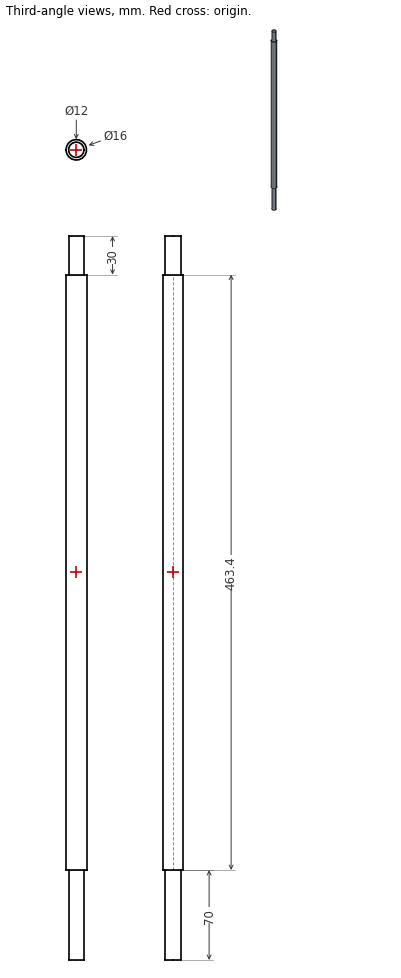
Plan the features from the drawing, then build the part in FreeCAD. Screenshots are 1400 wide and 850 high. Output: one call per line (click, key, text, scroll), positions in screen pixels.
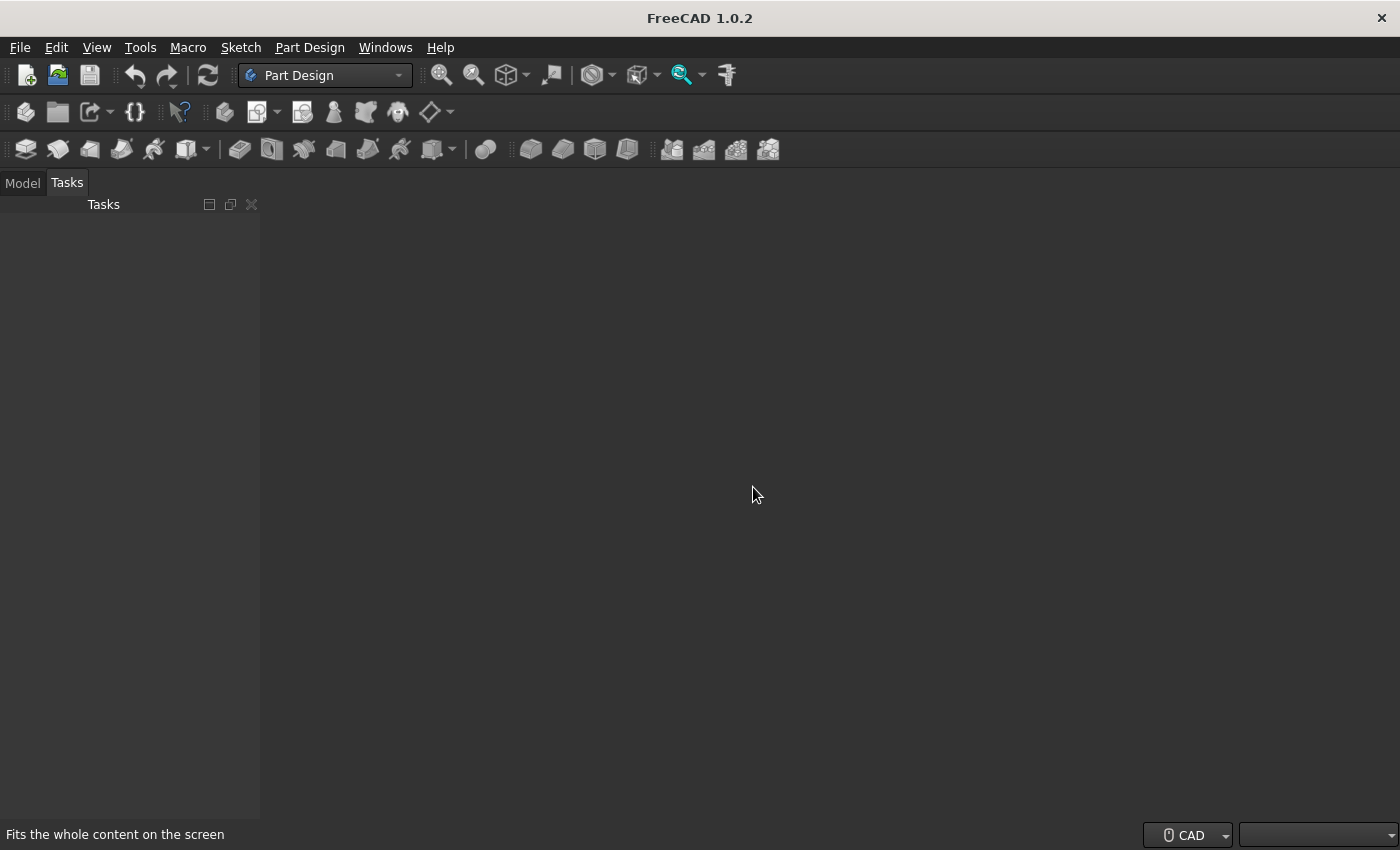
click(26, 76)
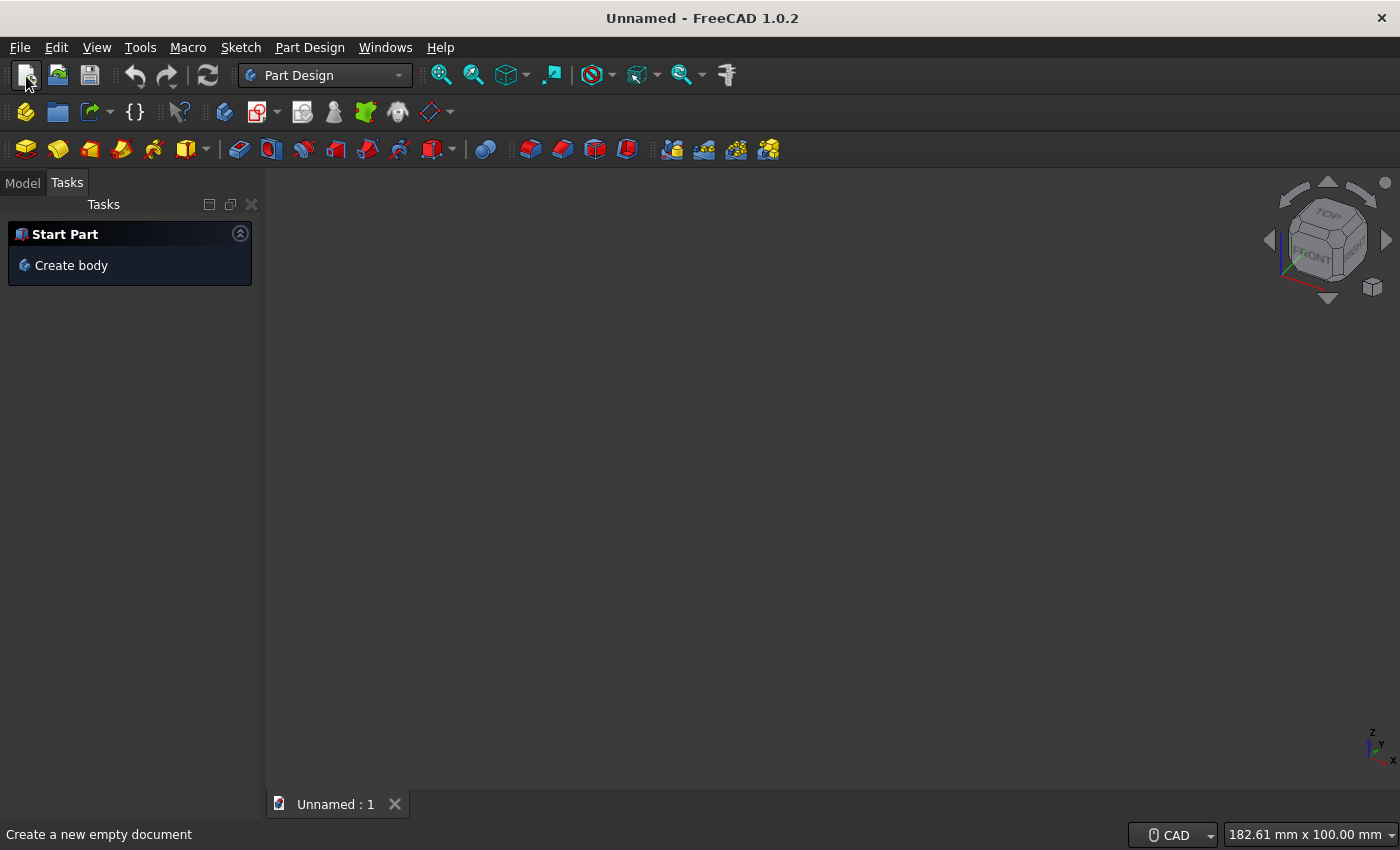
click(258, 112)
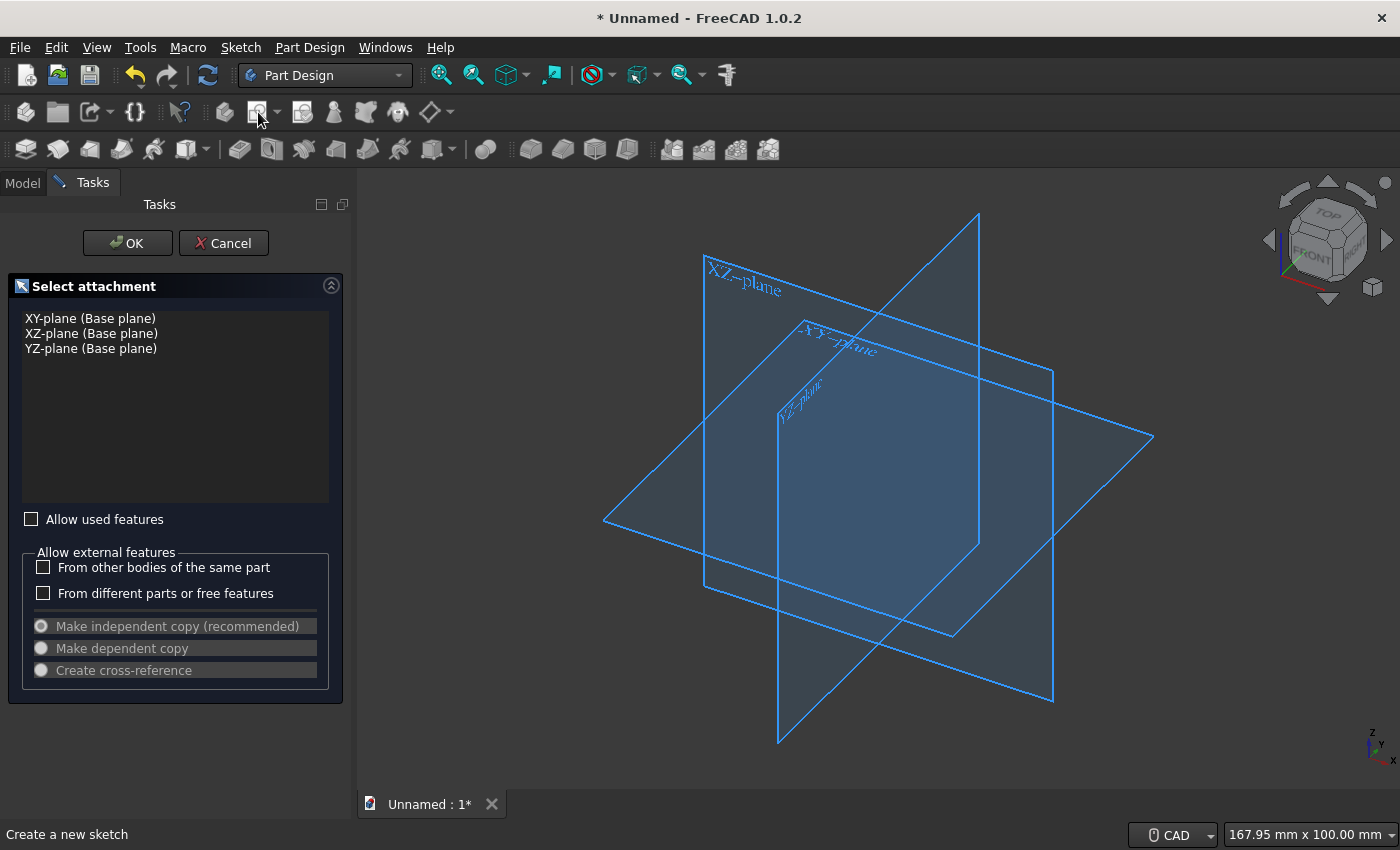
click(82, 318)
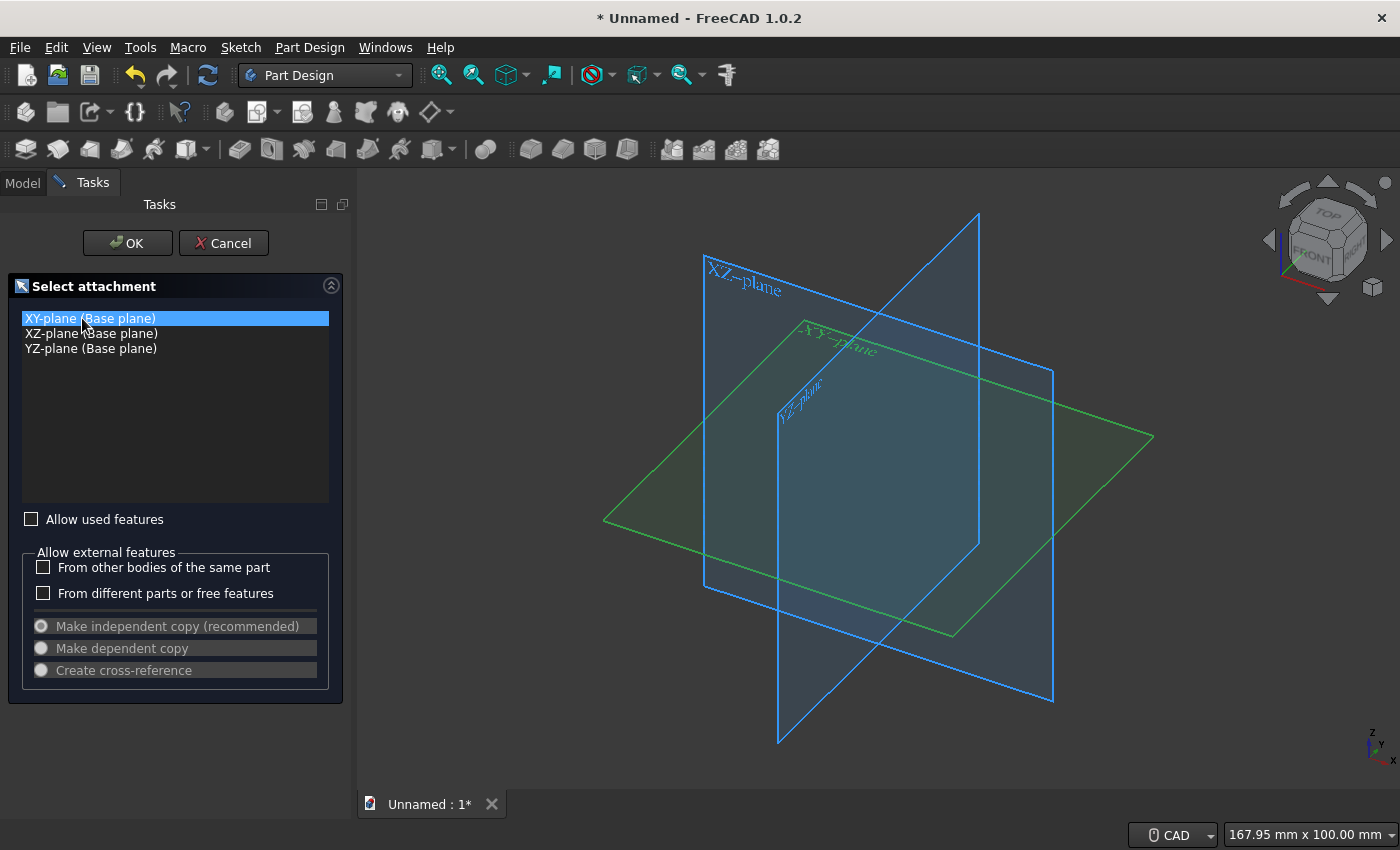
click(128, 243)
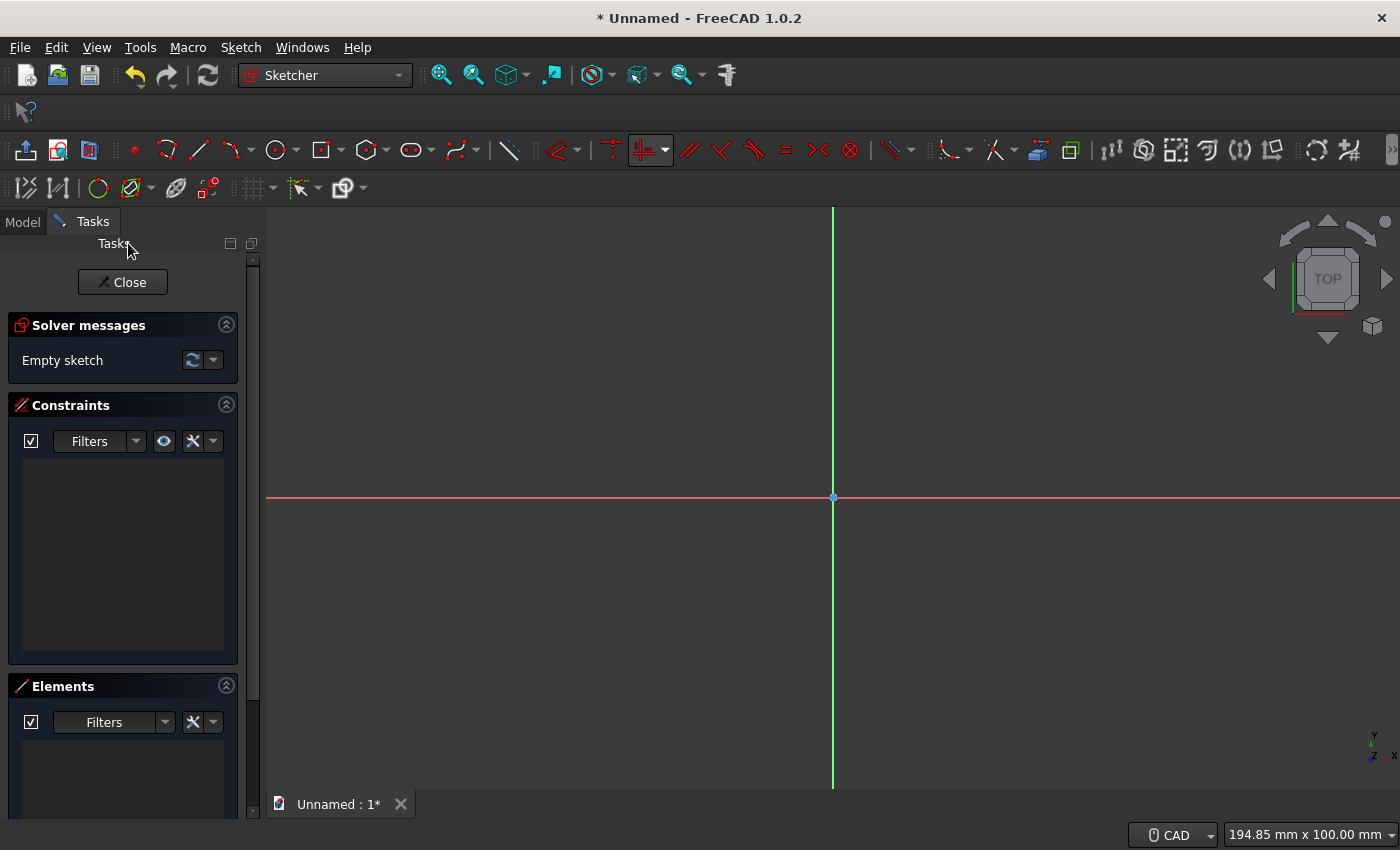
scroll(855, 498, up, 7)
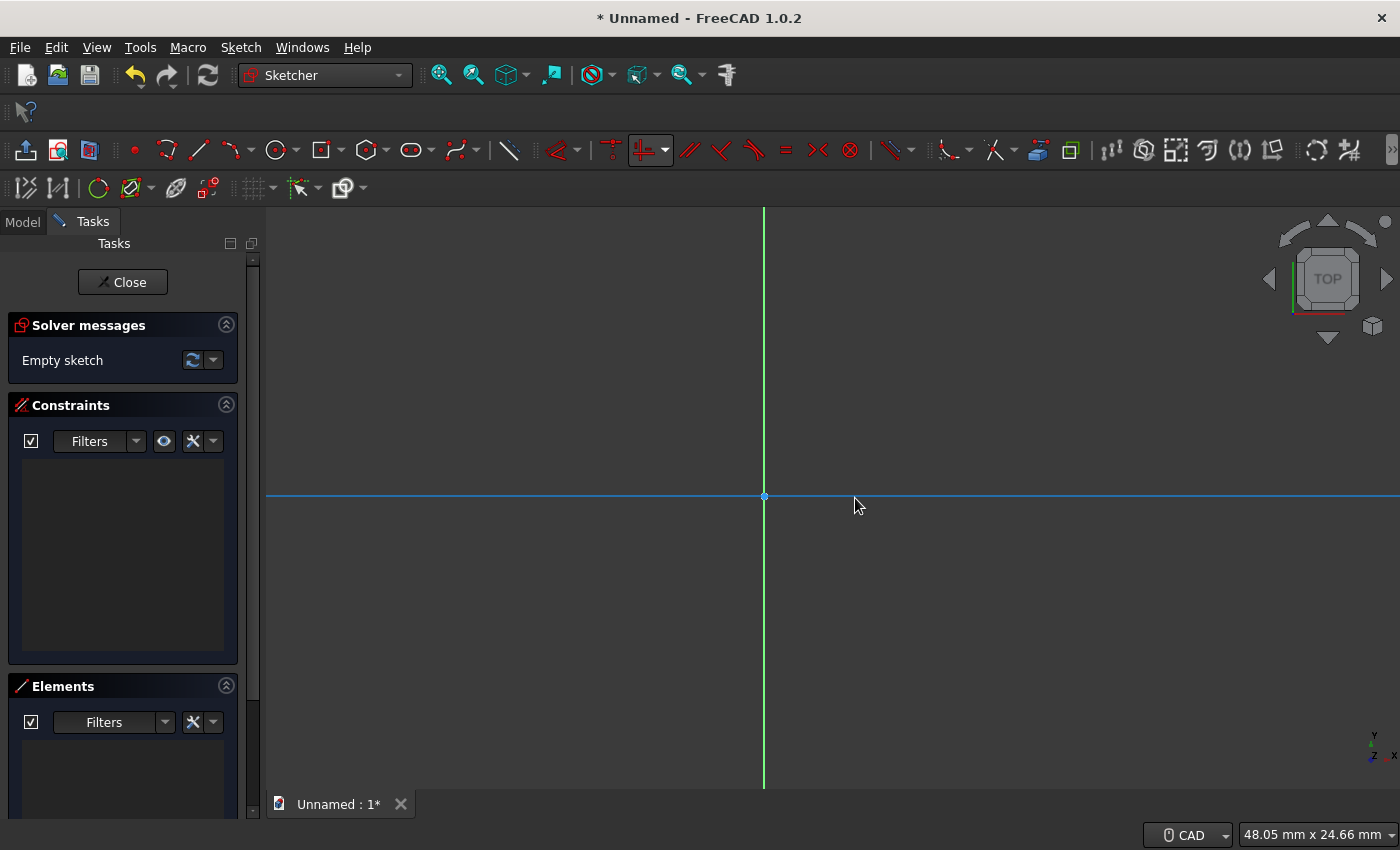
click(276, 150)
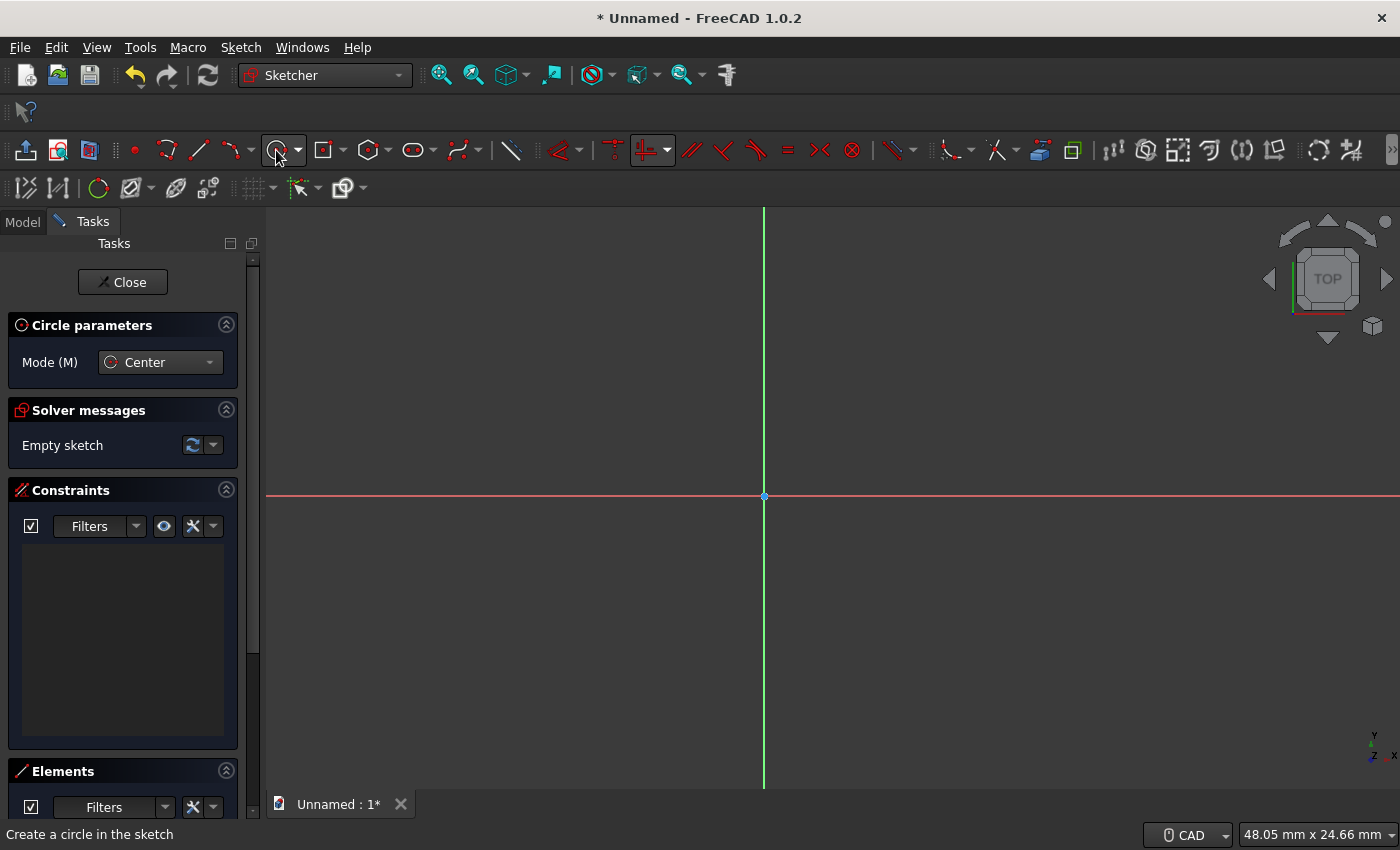
click(764, 496)
click(898, 363)
key(Escape)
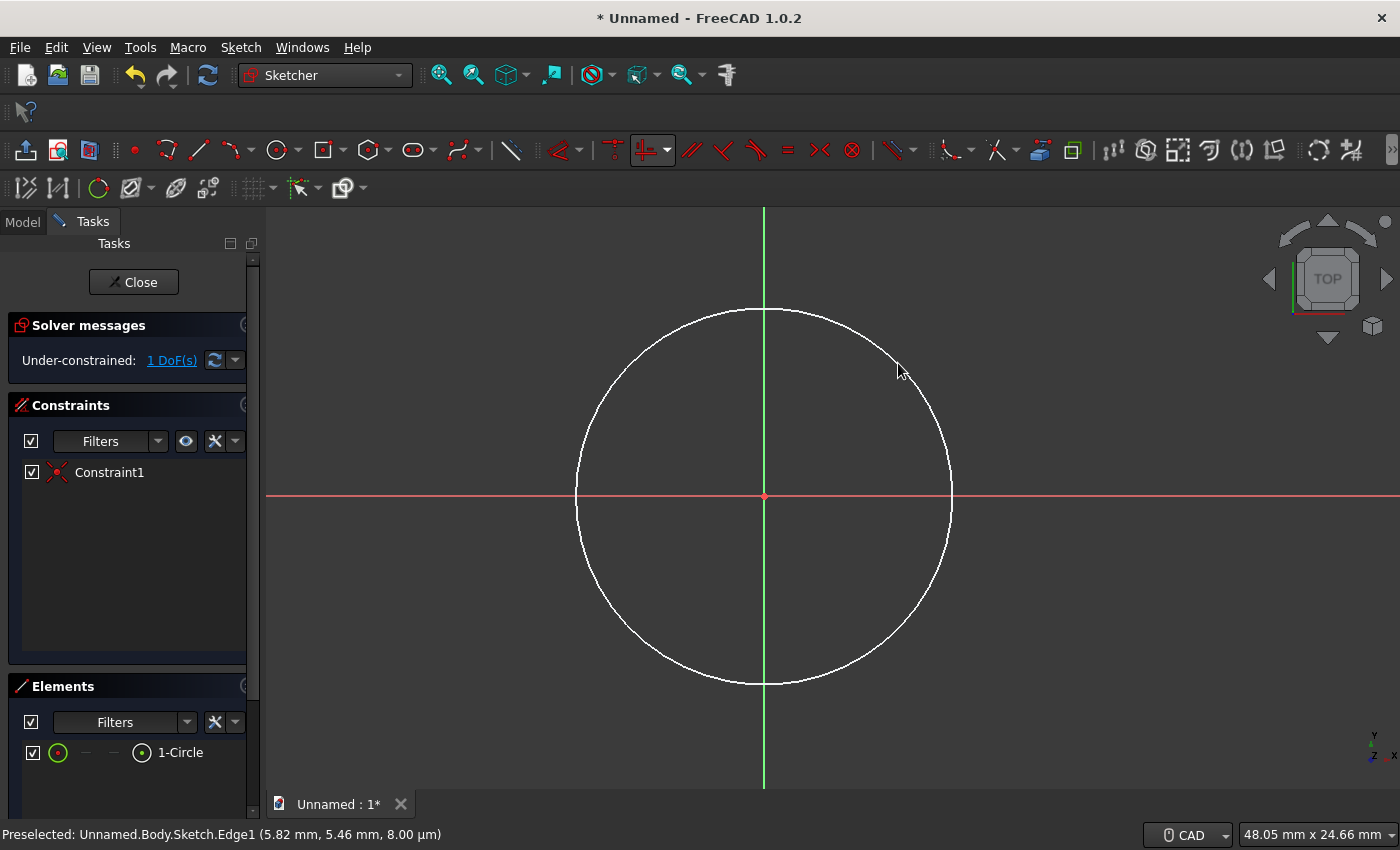
click(558, 150)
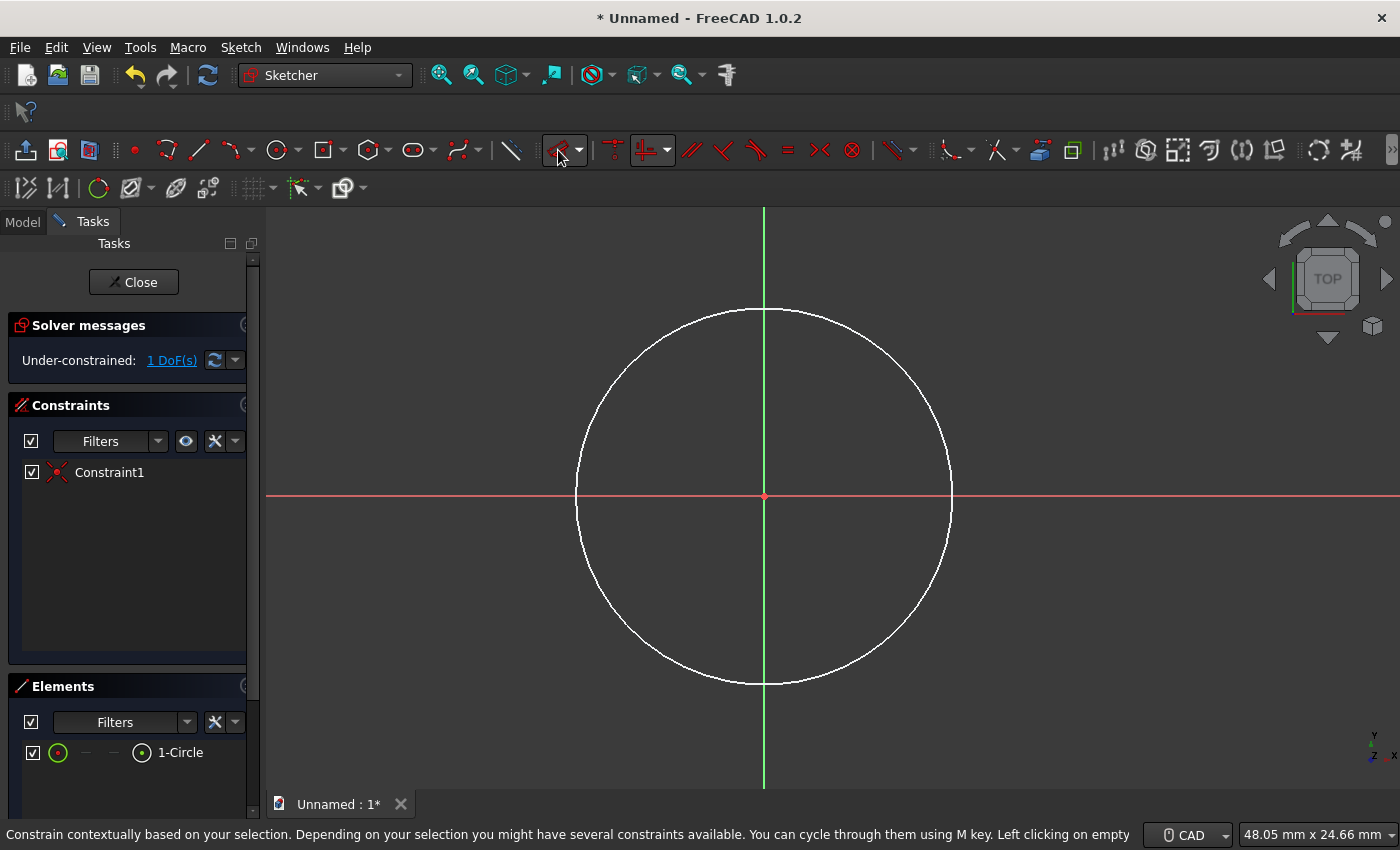
click(897, 363)
click(920, 340)